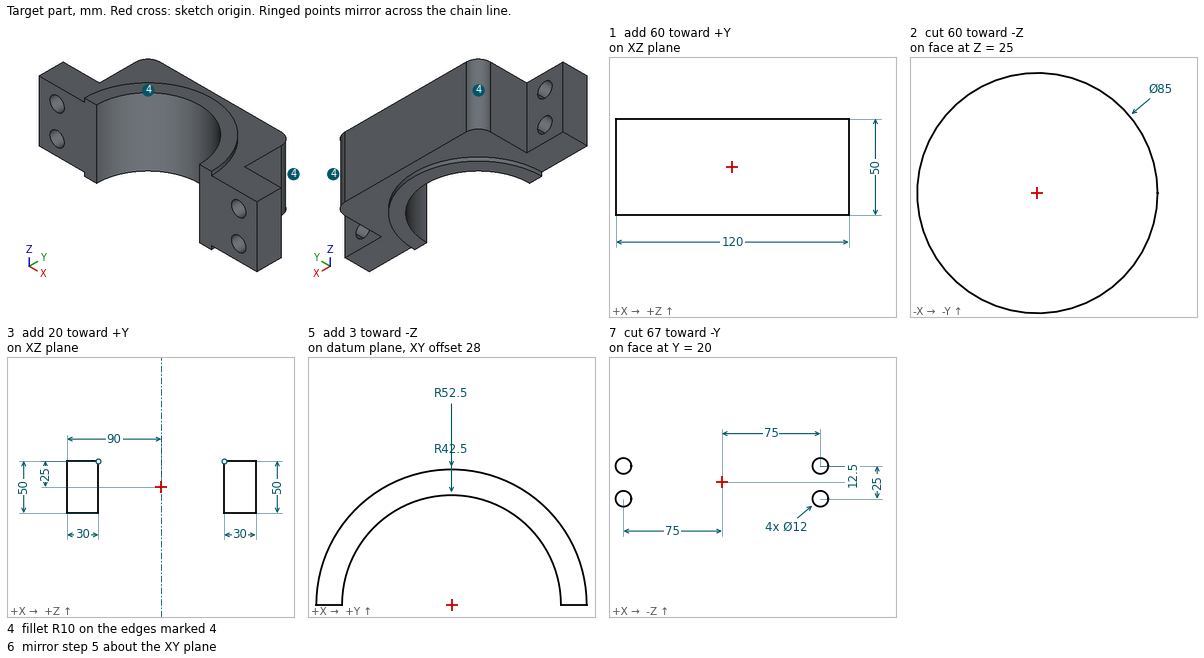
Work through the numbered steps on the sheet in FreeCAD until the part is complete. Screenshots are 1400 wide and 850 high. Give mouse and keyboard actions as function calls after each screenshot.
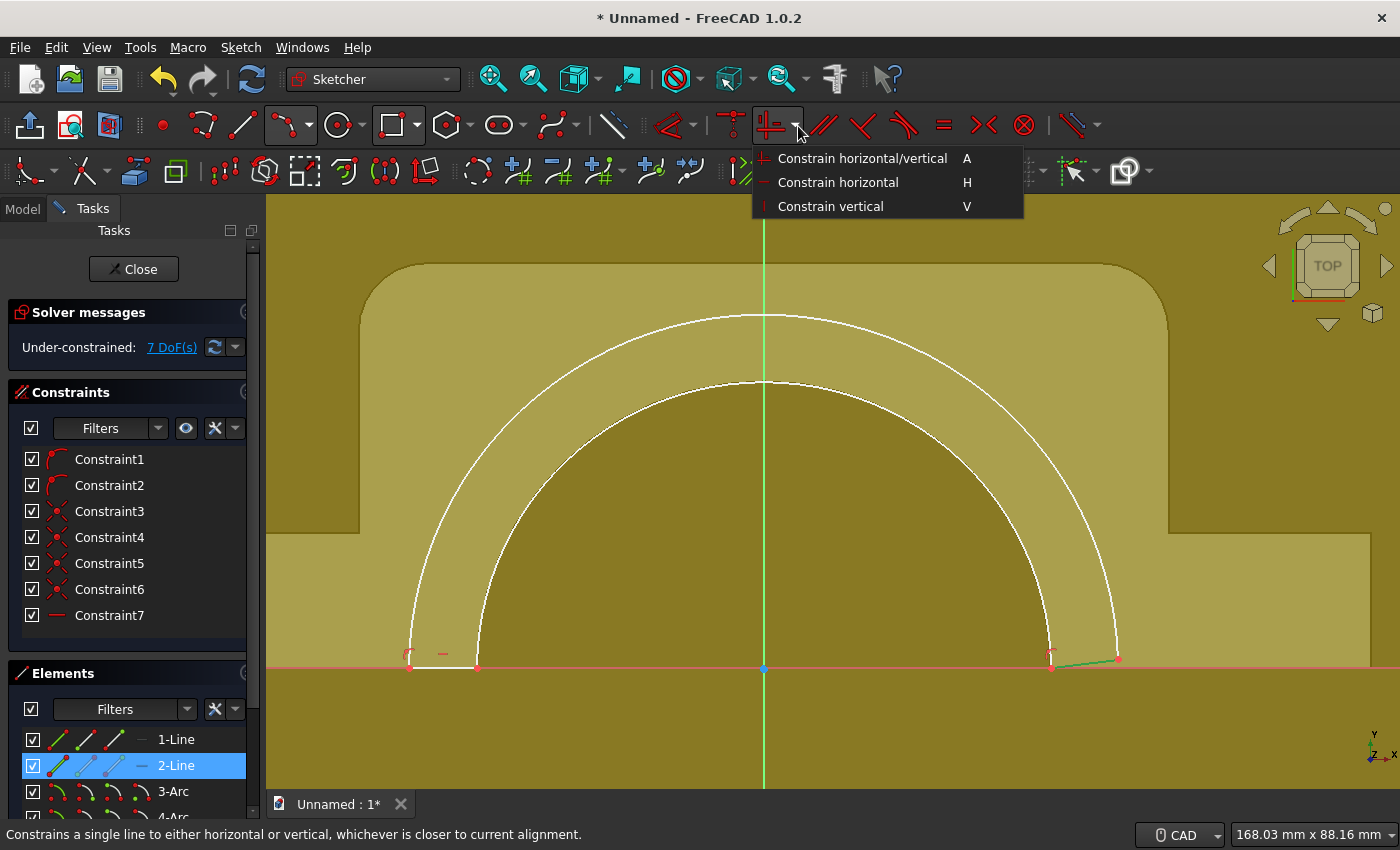
click(888, 182)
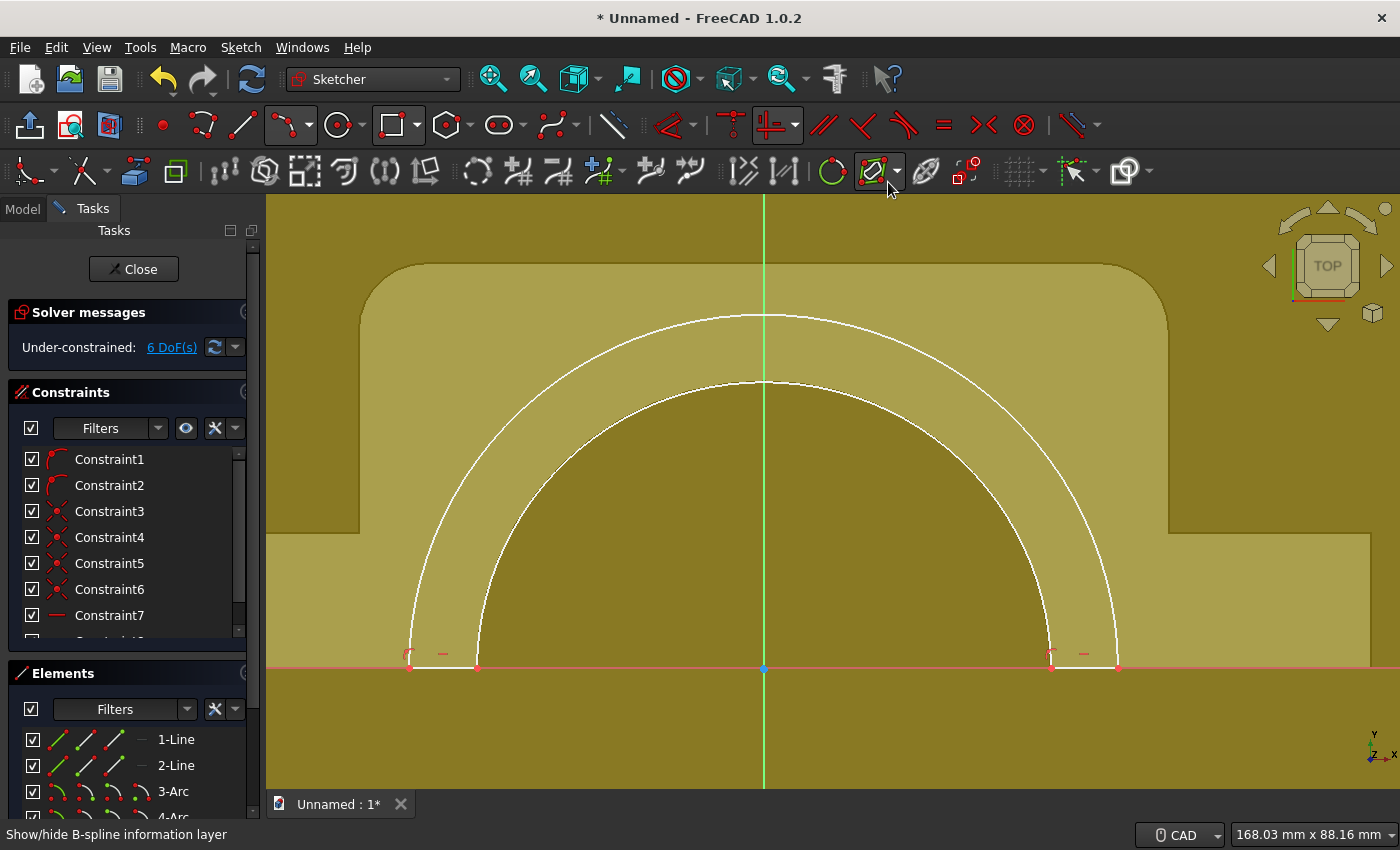
click(932, 437)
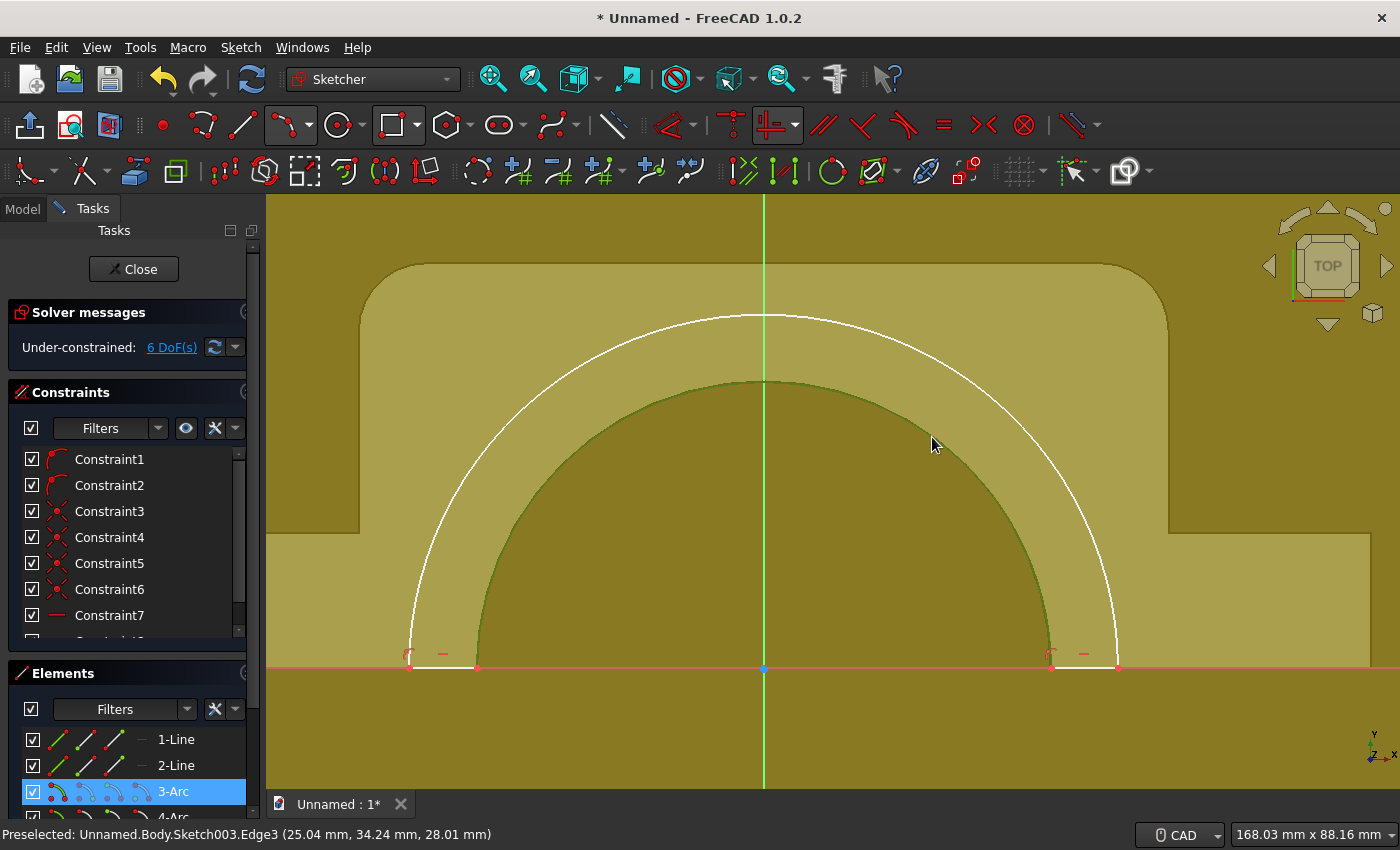
click(972, 382)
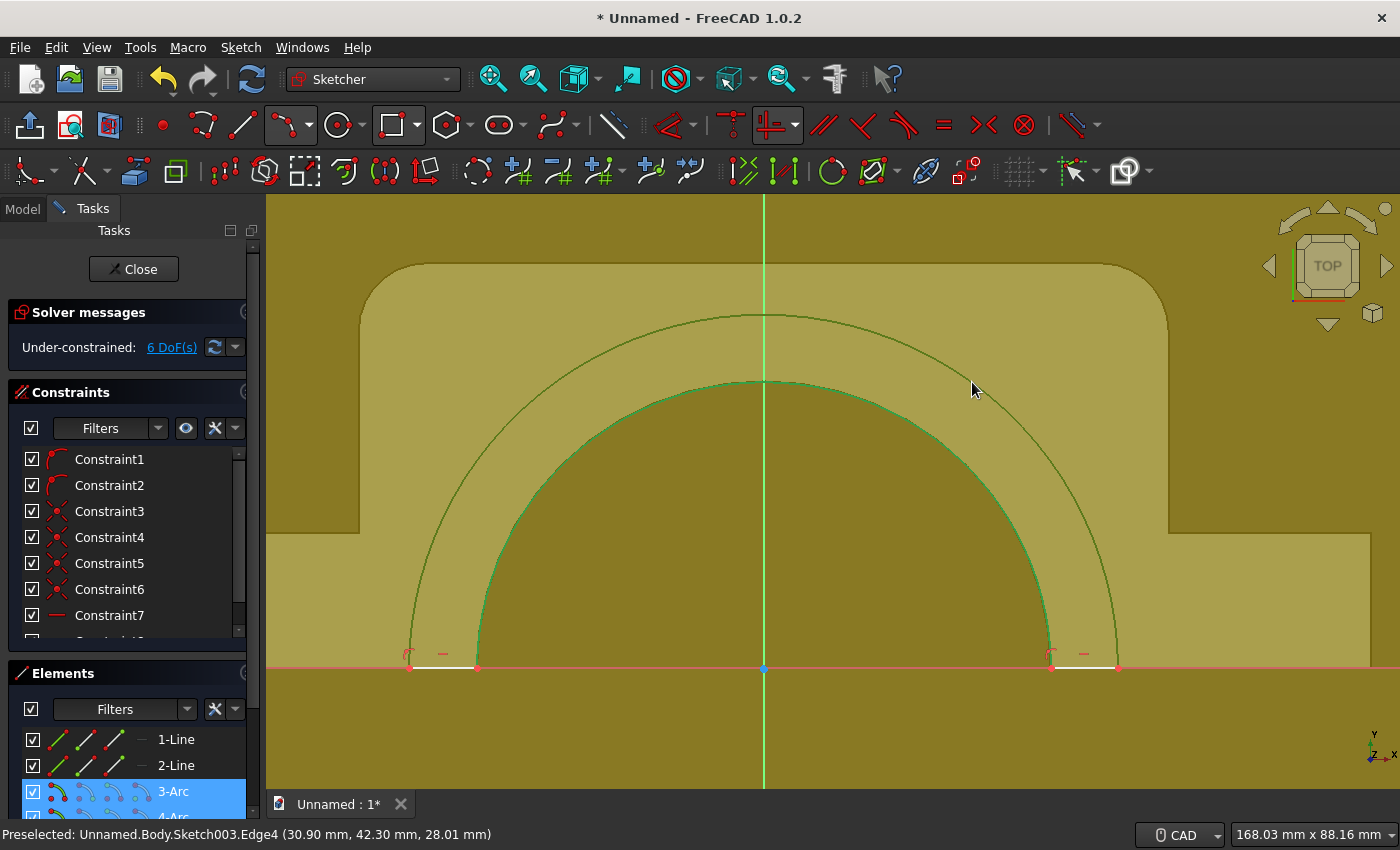
click(732, 126)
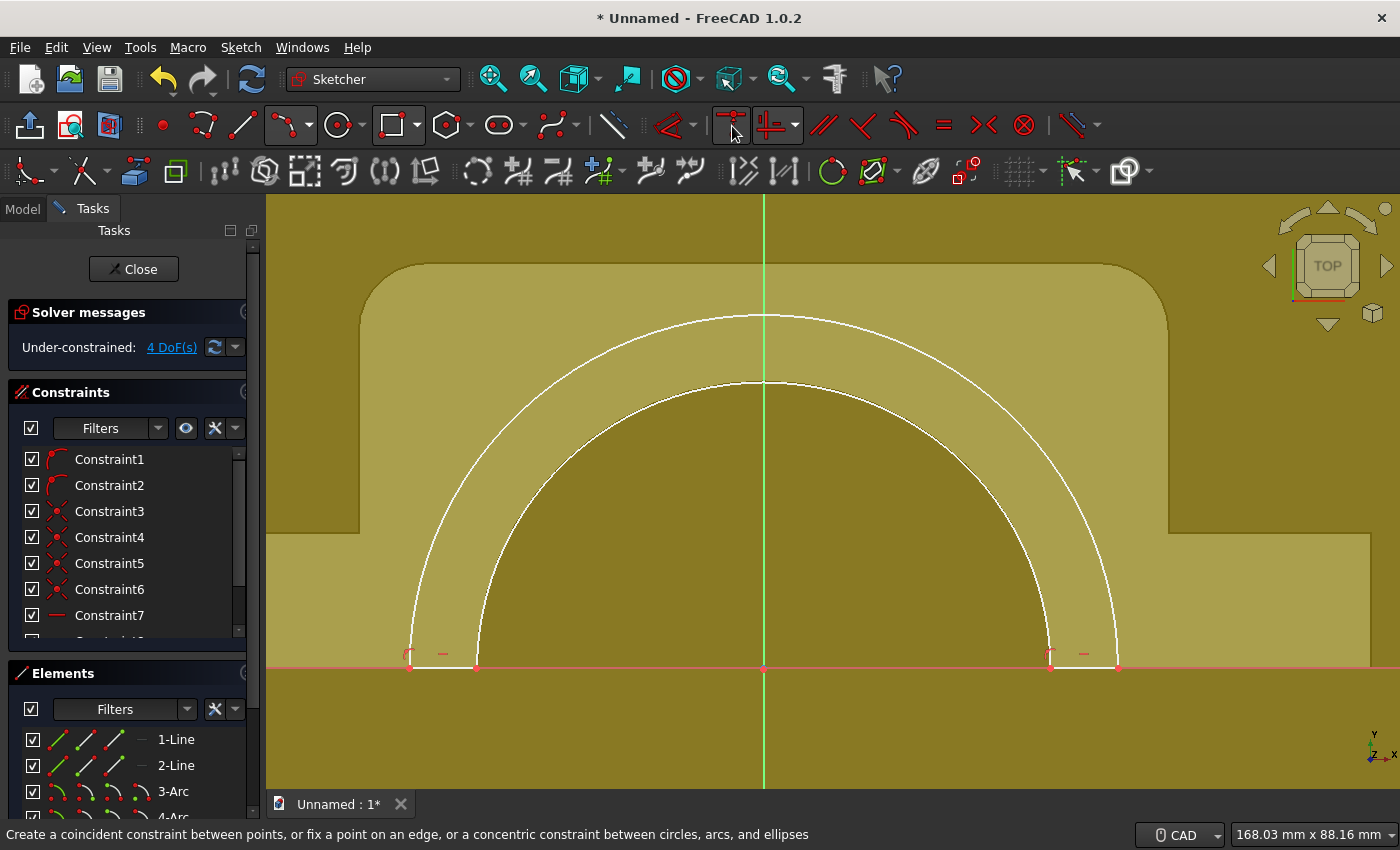
drag(754, 658, 774, 679)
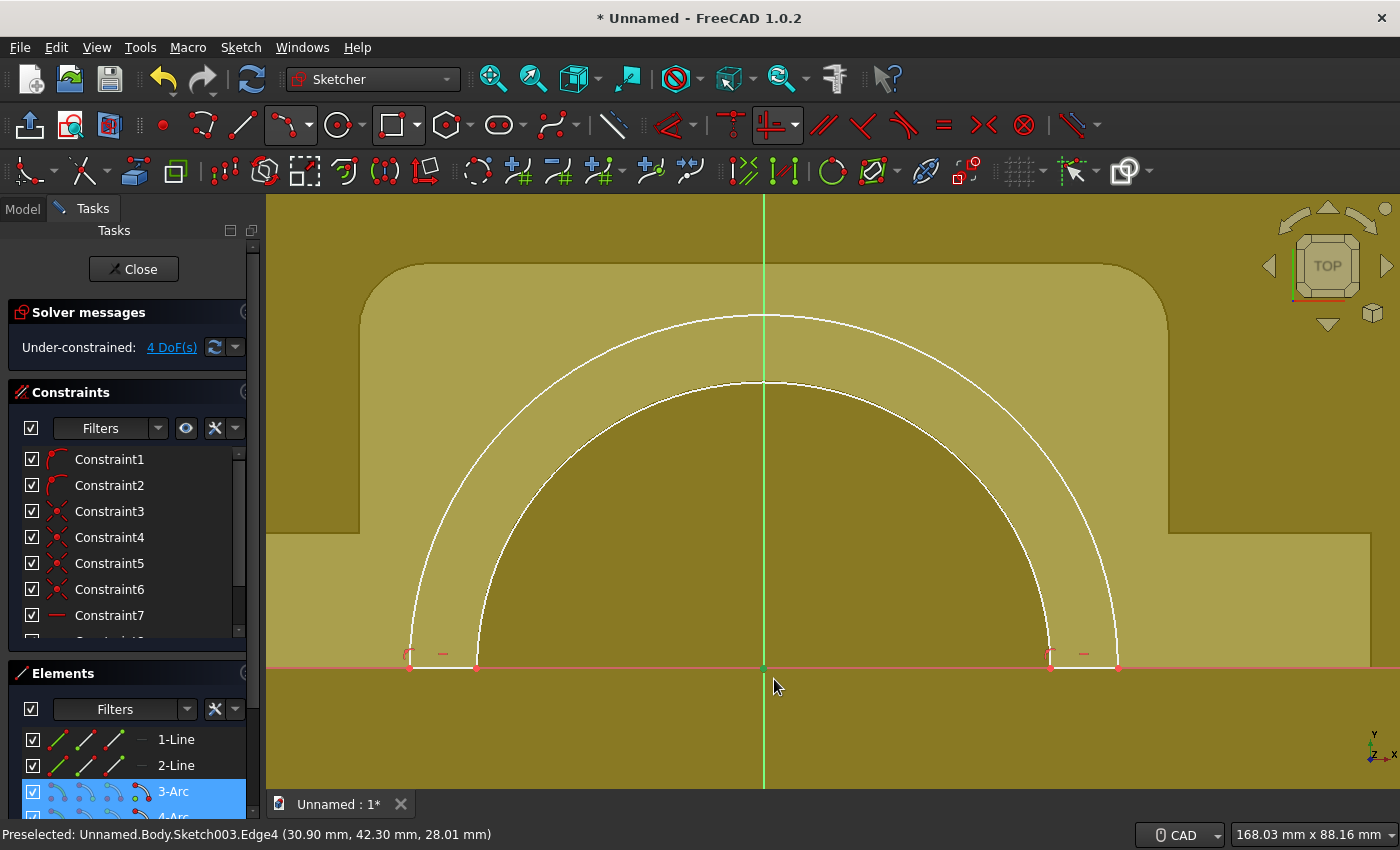
click(732, 126)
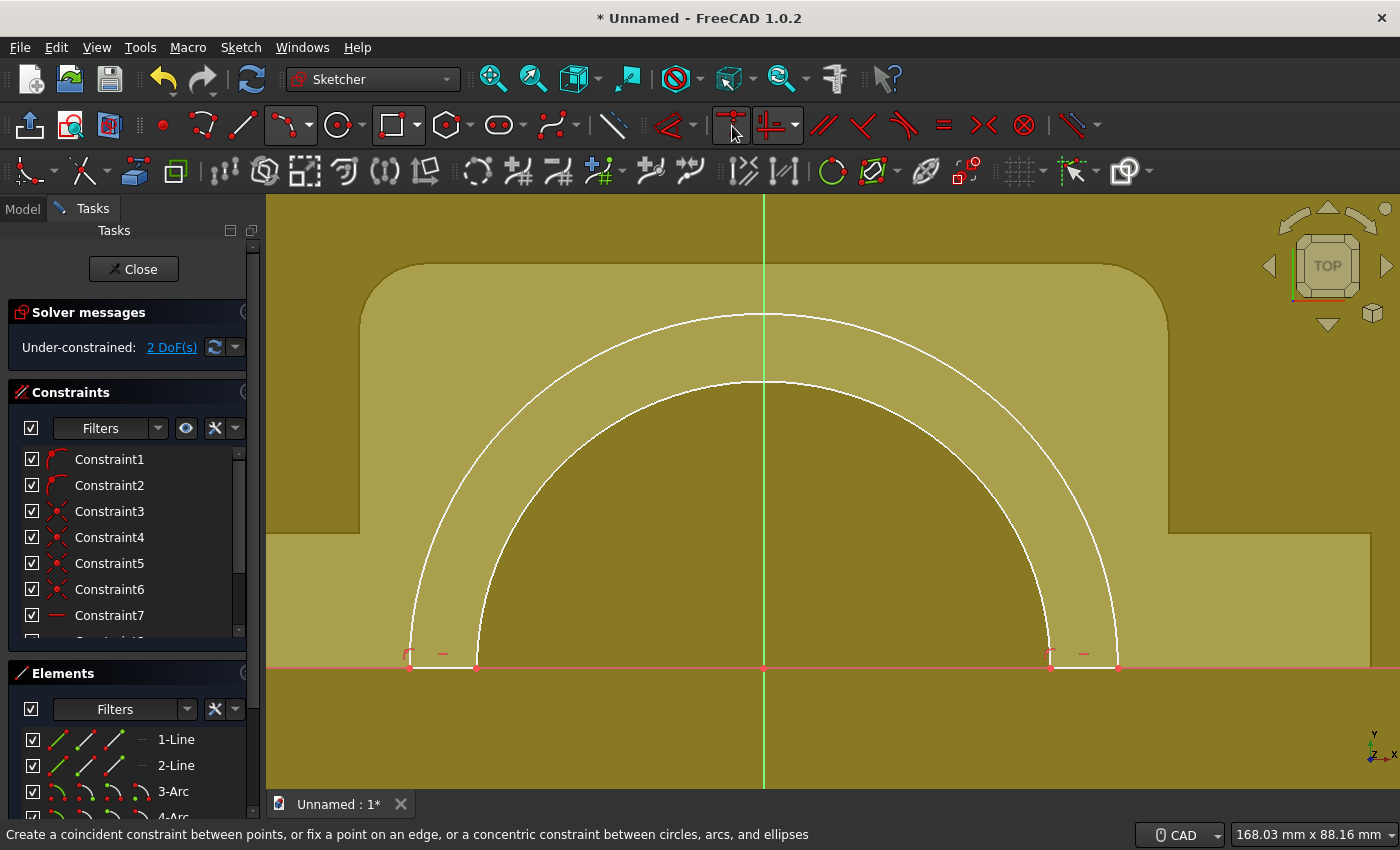
click(668, 126)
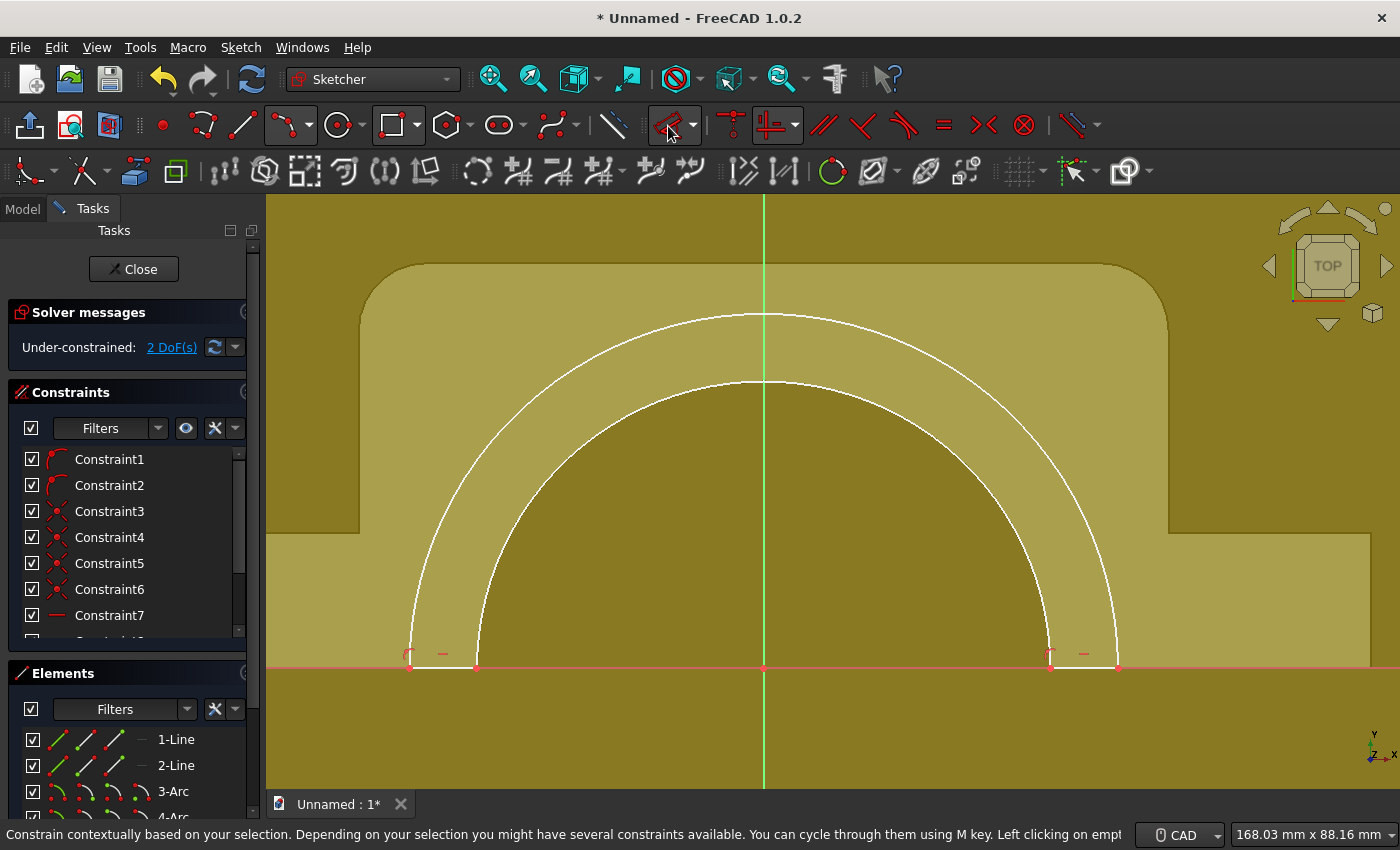
click(932, 436)
click(951, 410)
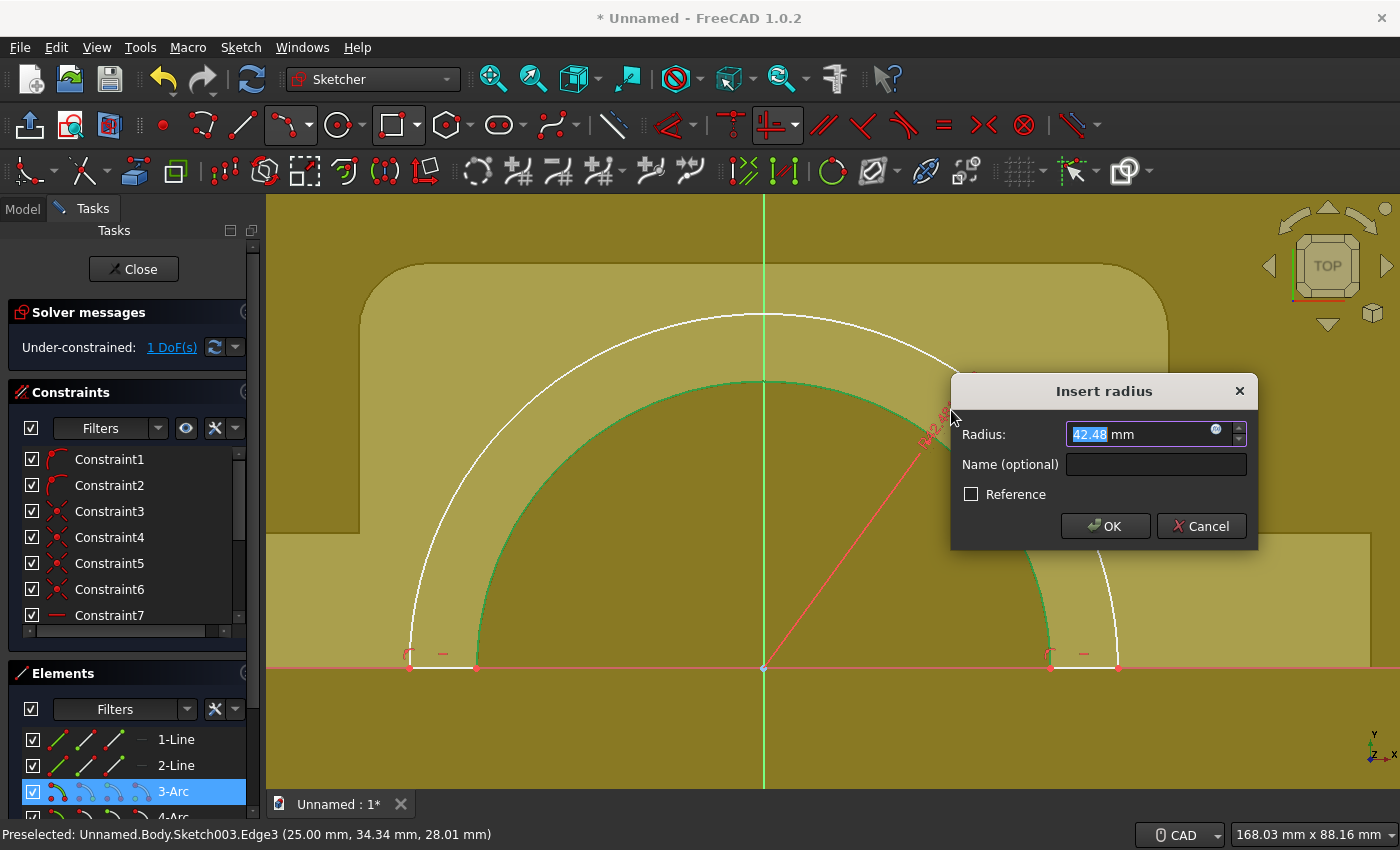
text(42.5)
key(Return)